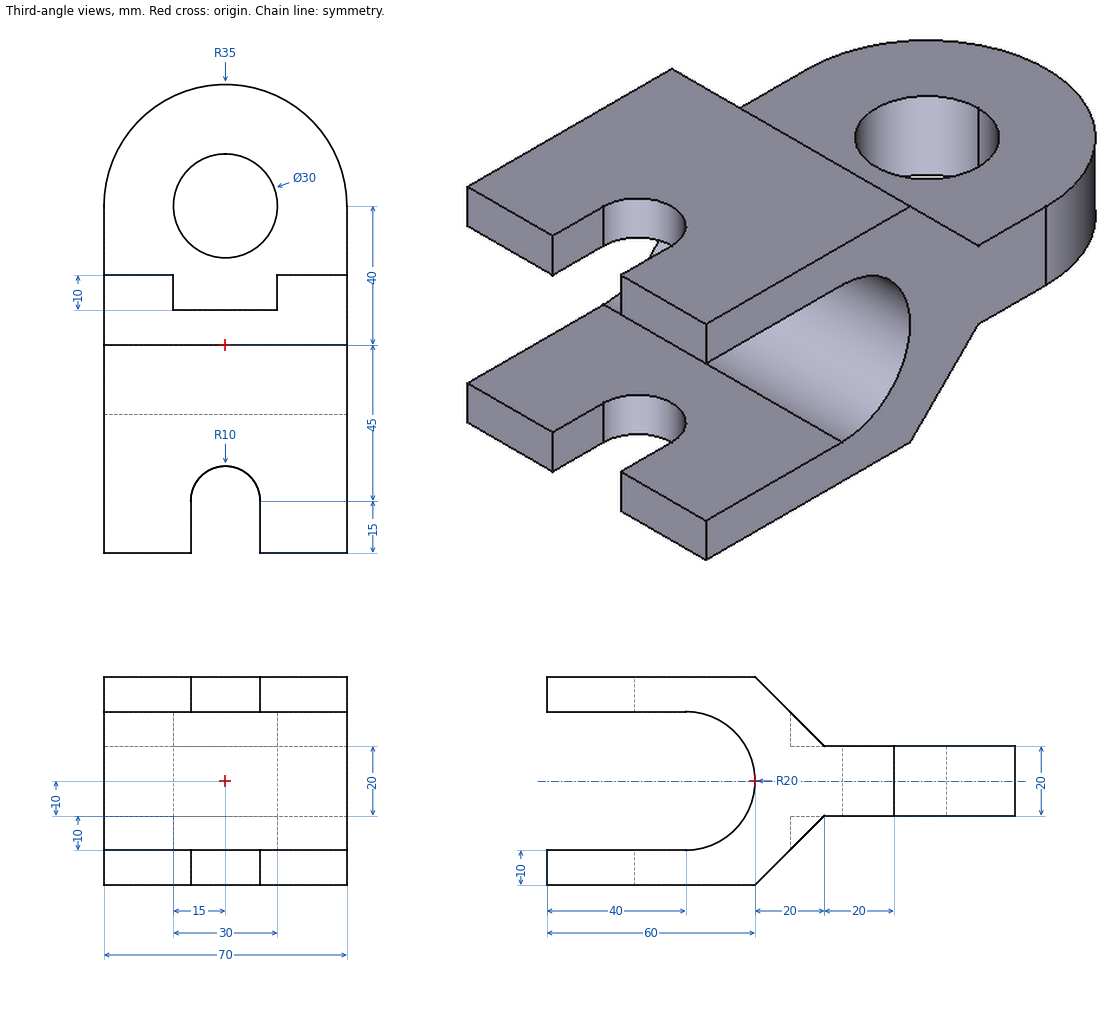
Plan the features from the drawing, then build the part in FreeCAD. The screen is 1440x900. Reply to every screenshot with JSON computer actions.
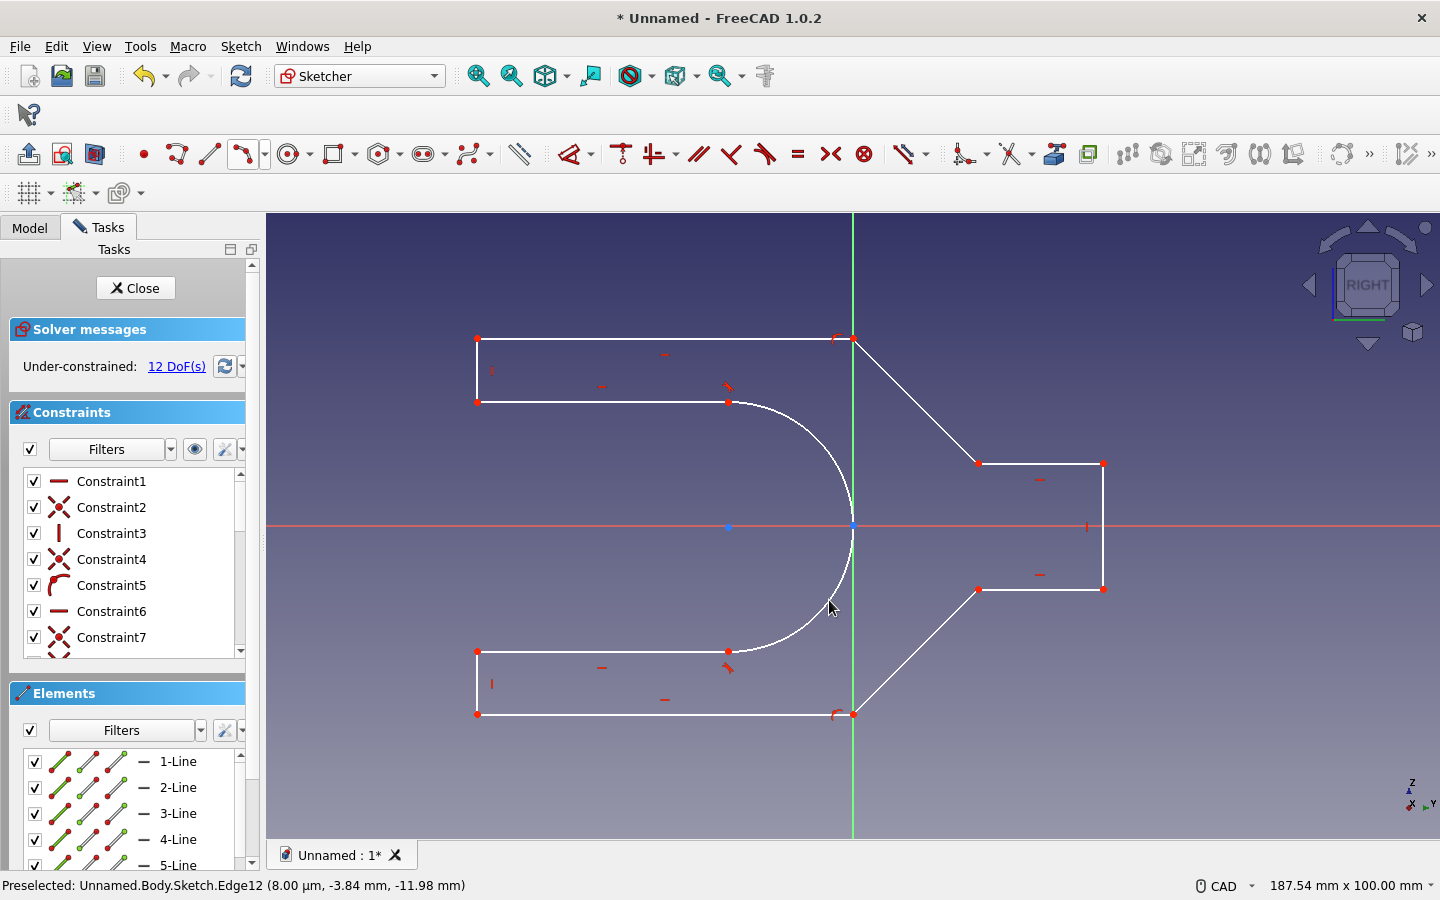
{"action": "left_click", "coordinate": [728, 527]}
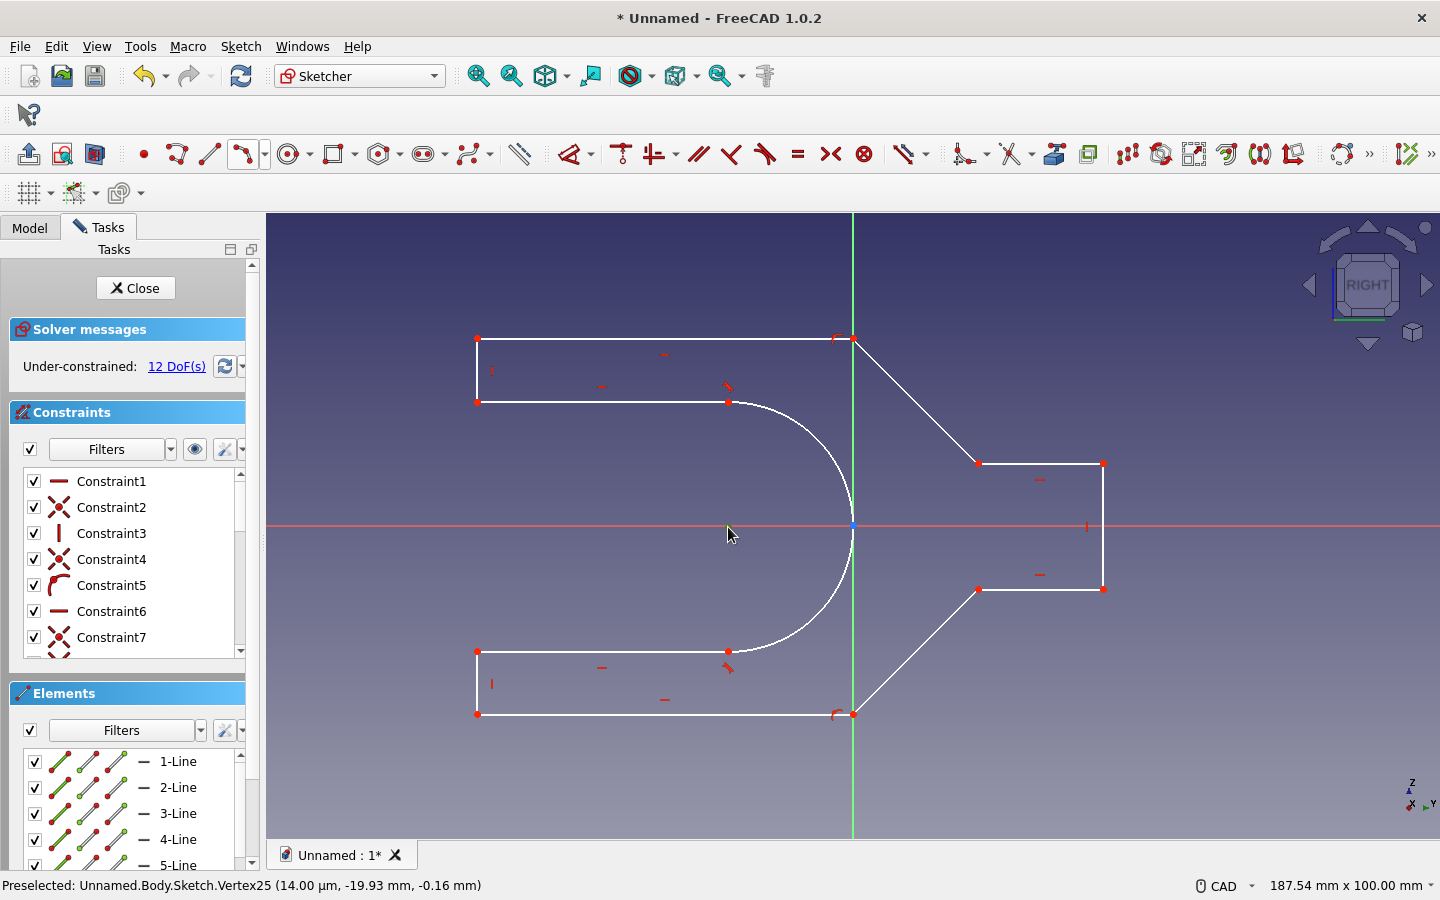
{"action": "left_click", "coordinate": [364, 526]}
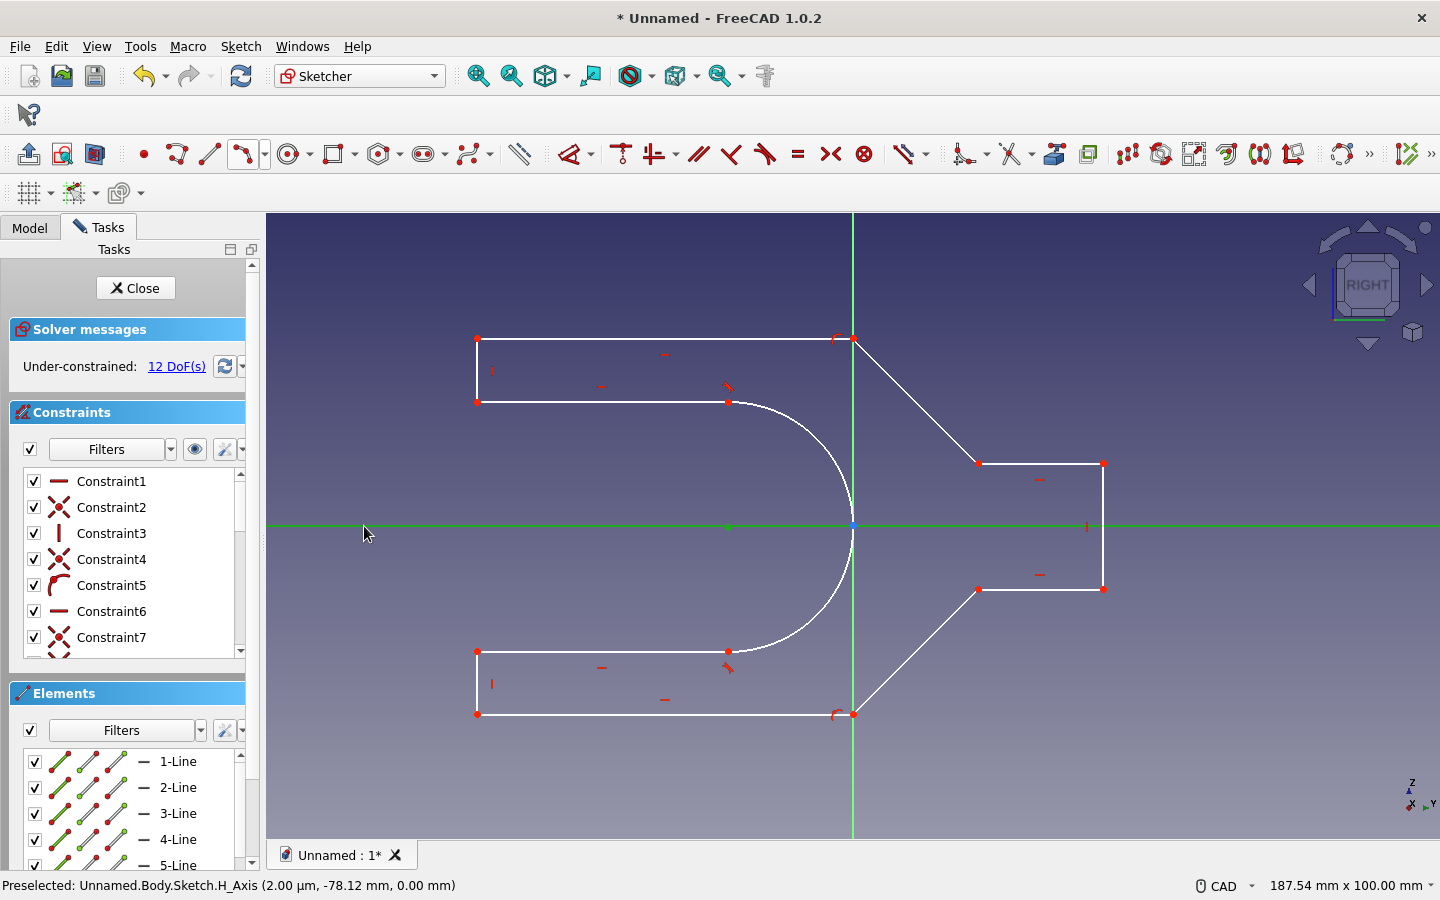
{"action": "key", "text": "c"}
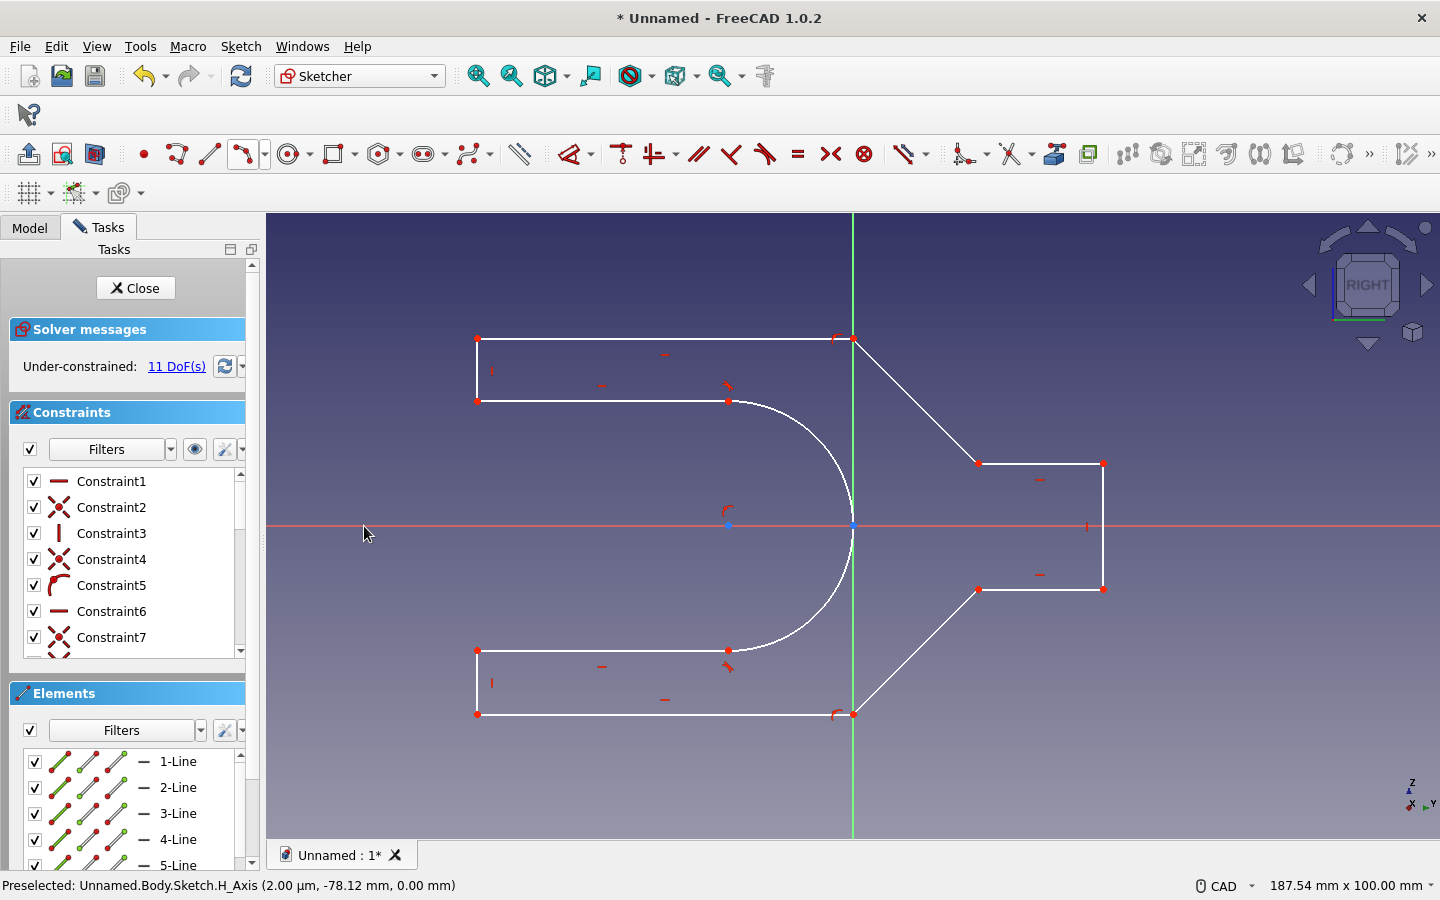
{"action": "left_click", "coordinate": [978, 590]}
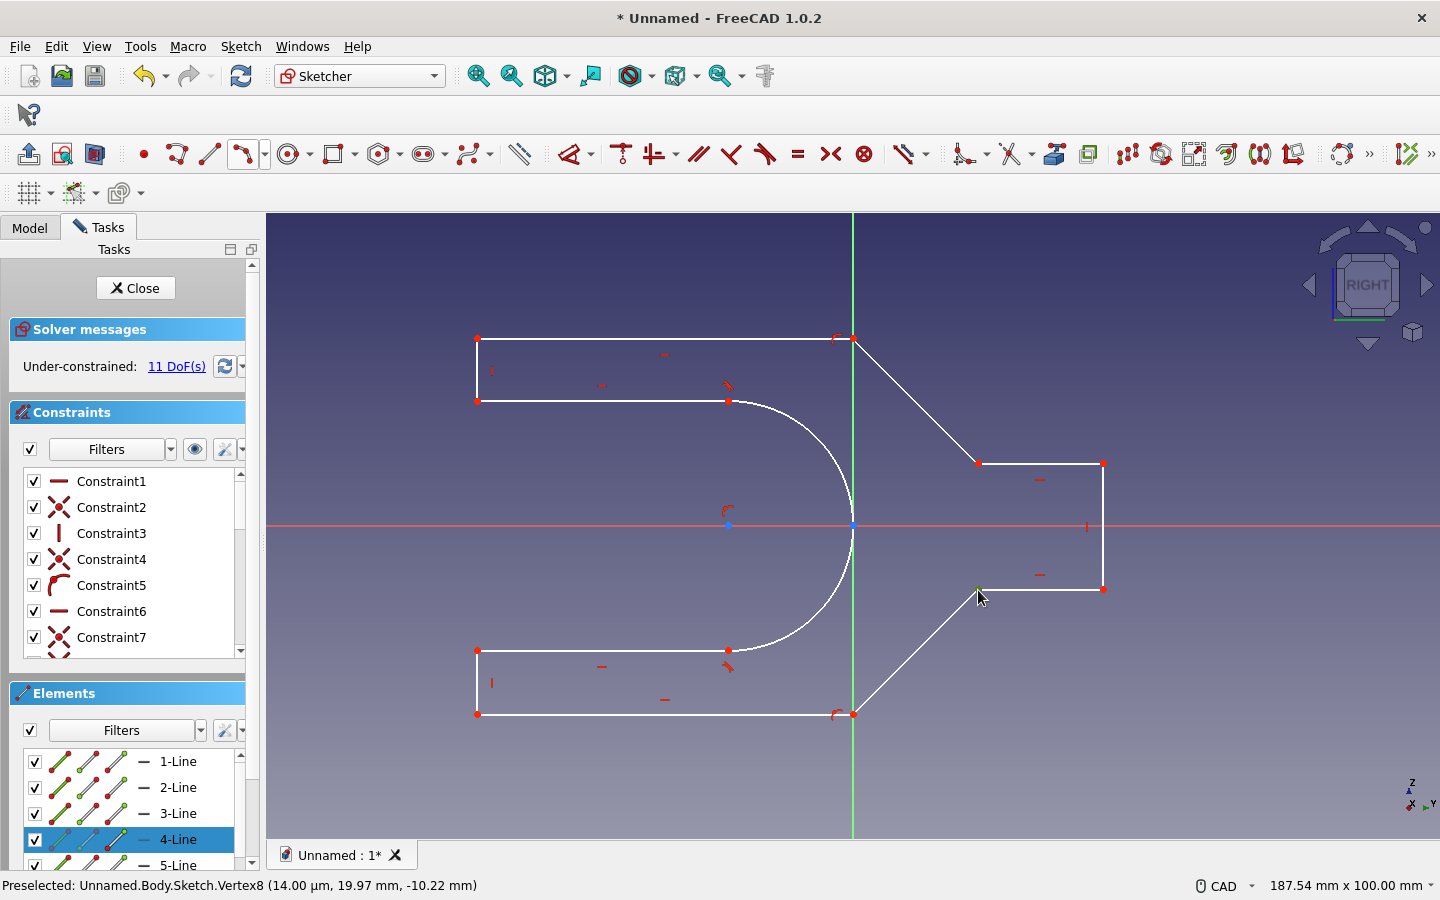
{"action": "left_click", "coordinate": [978, 464]}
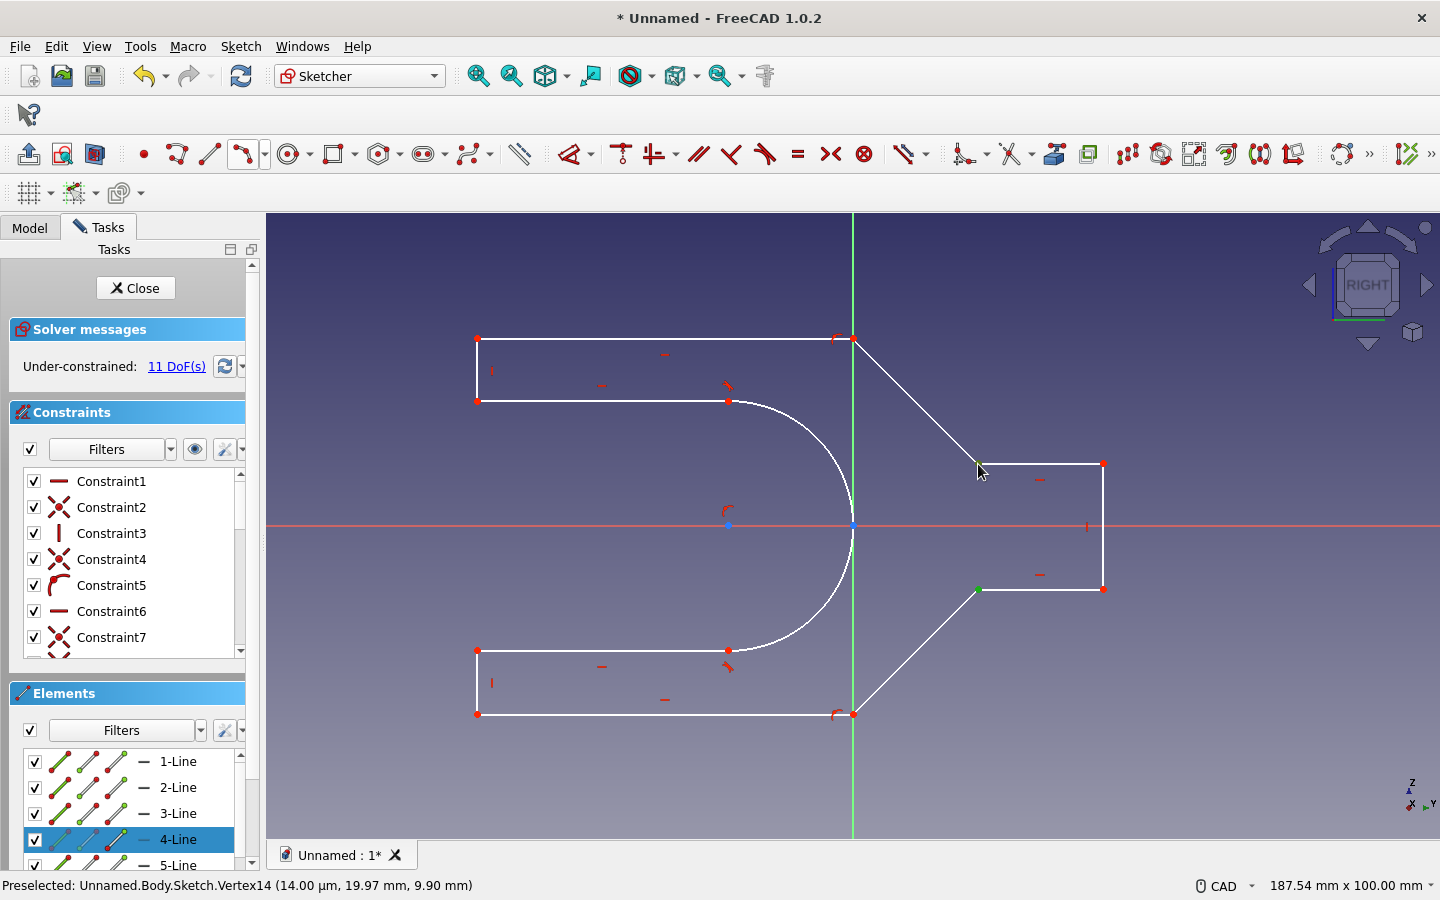
{"action": "left_click", "coordinate": [364, 526]}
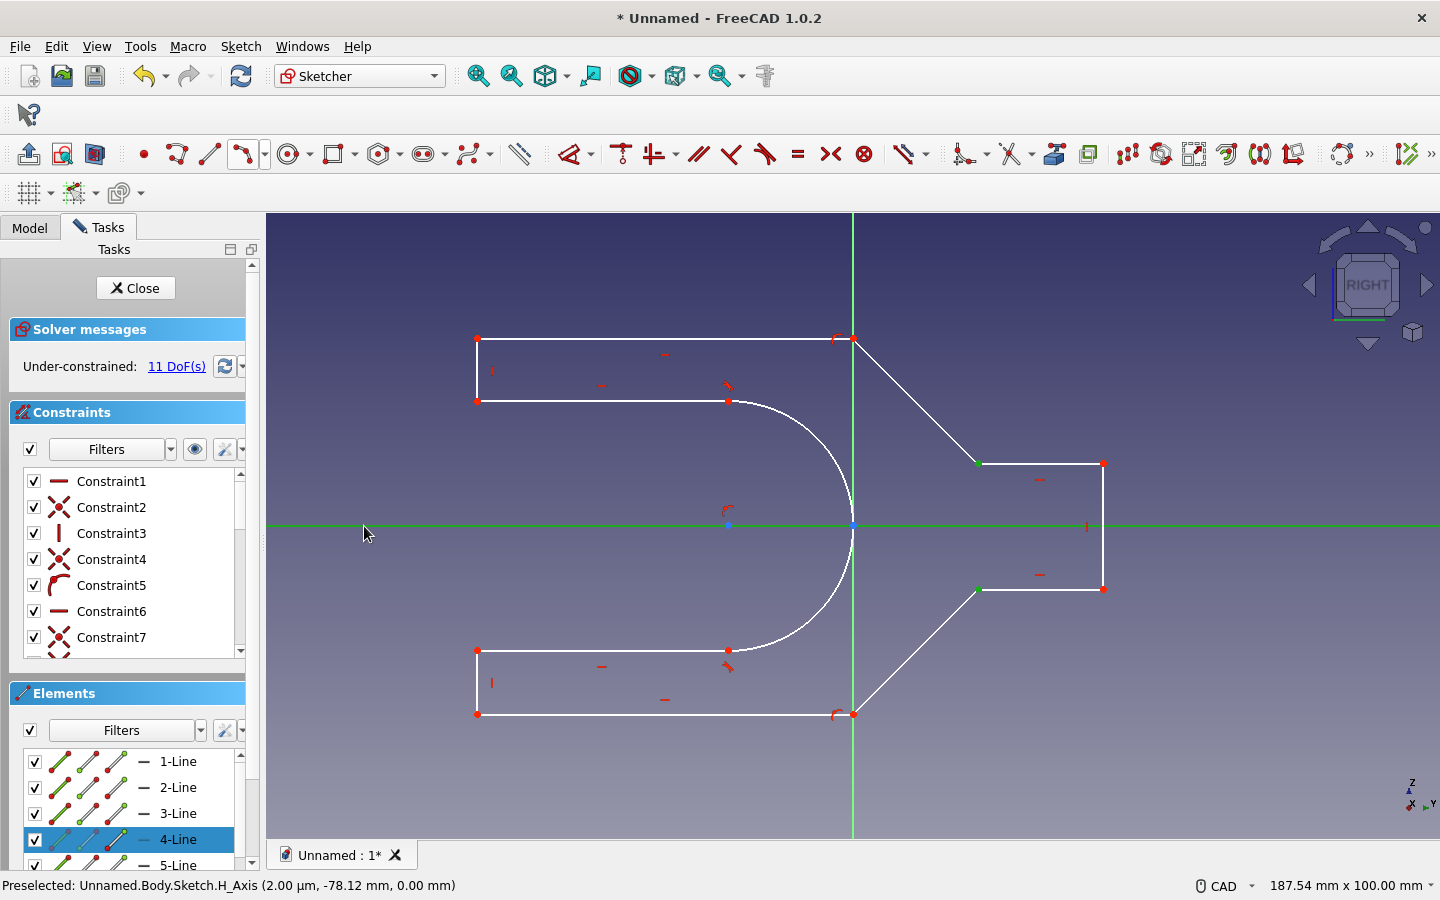
{"action": "key", "text": "s"}